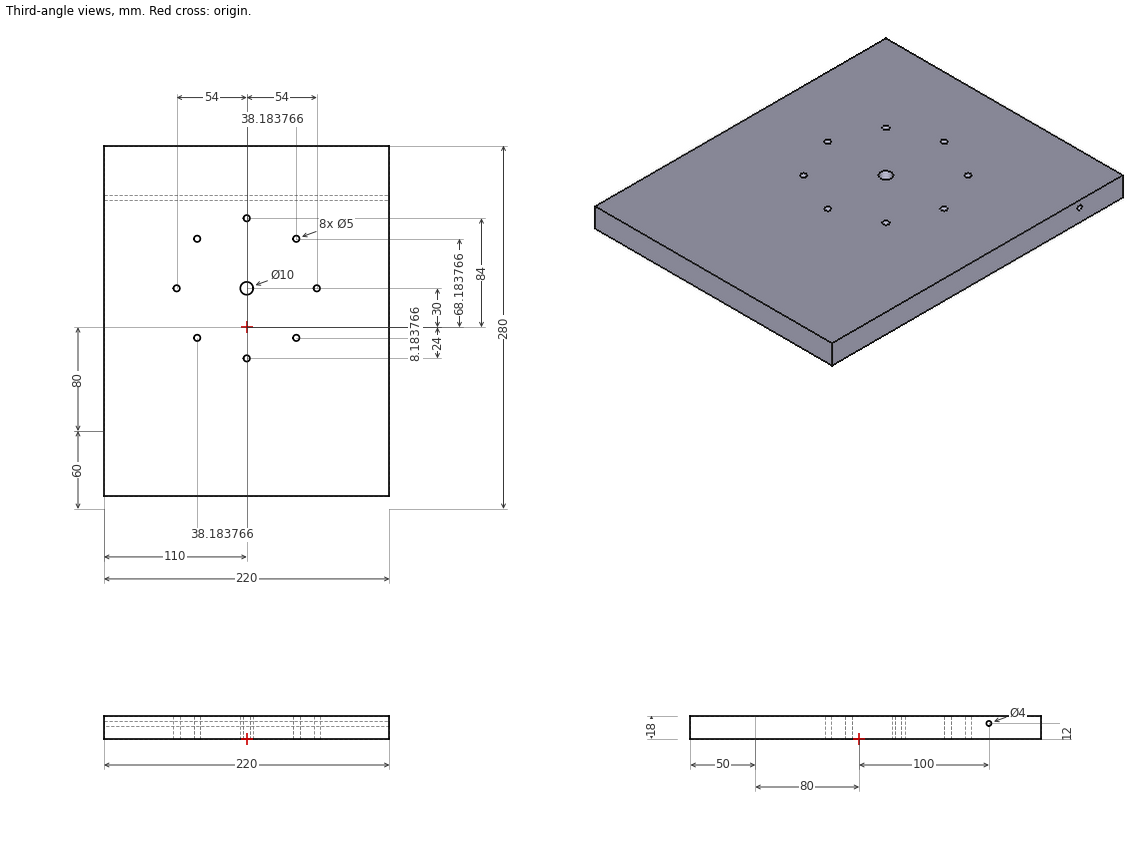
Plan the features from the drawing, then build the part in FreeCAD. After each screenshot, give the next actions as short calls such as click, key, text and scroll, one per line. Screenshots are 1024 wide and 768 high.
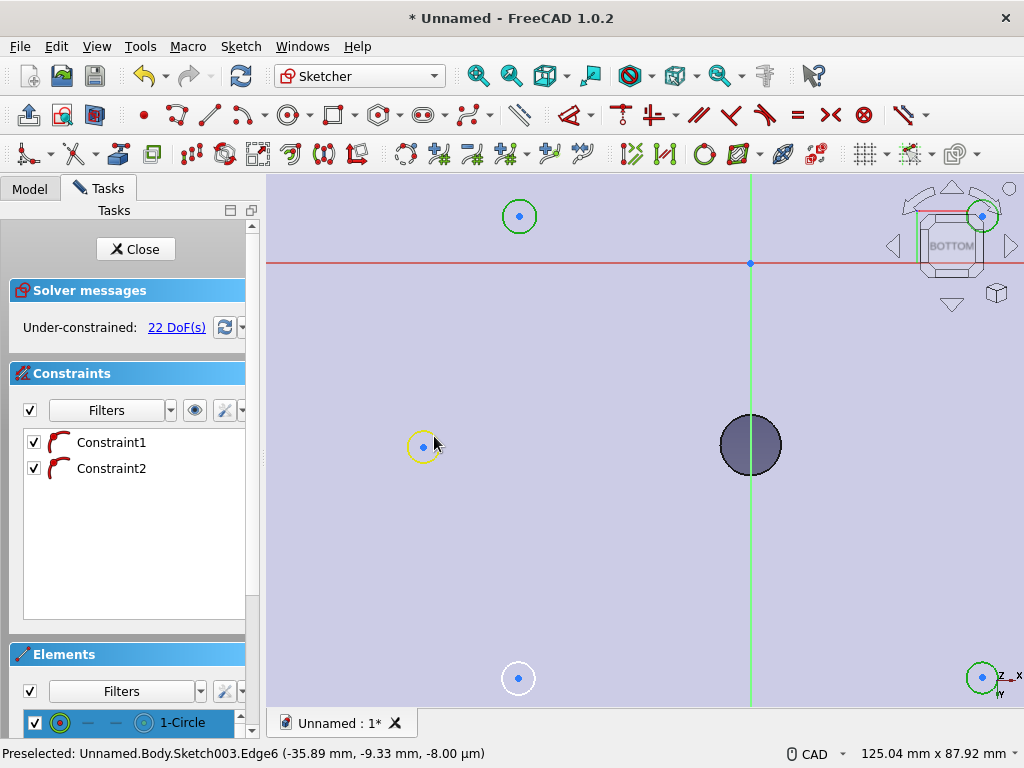
click(435, 436)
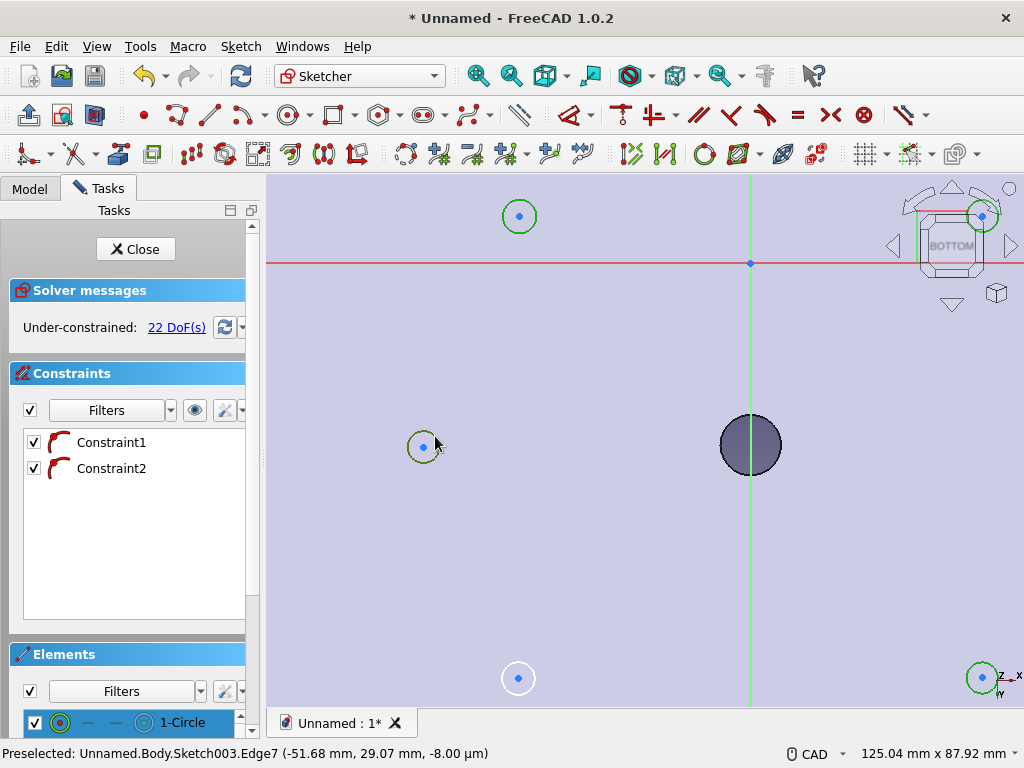
click(530, 667)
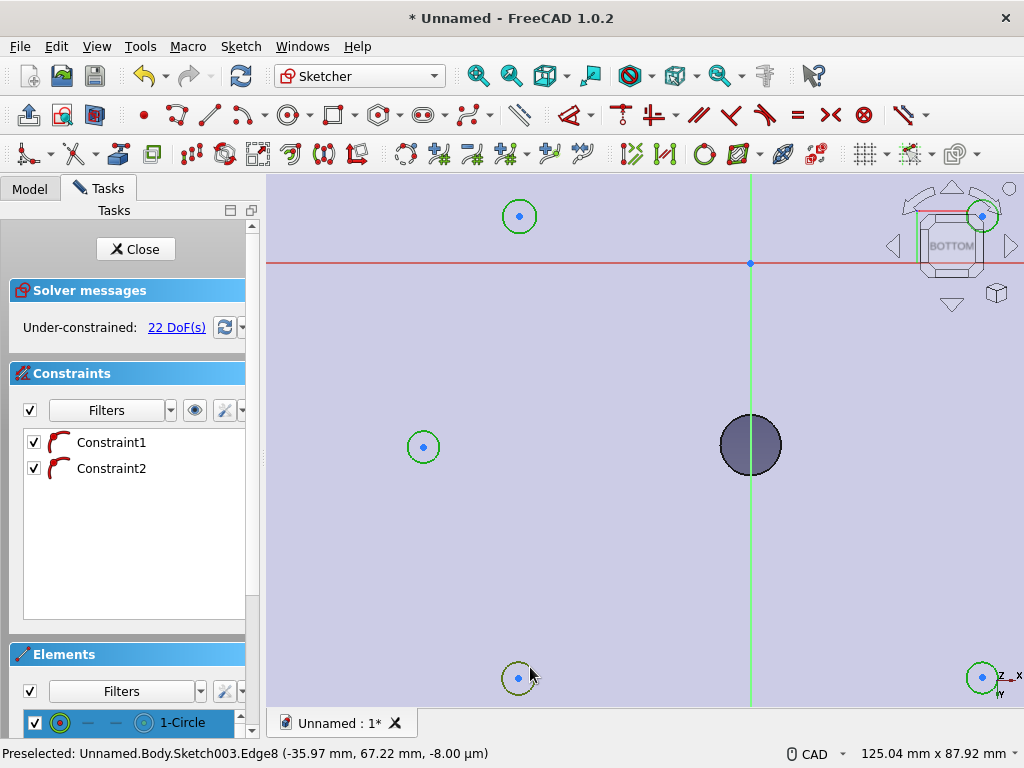
click(798, 116)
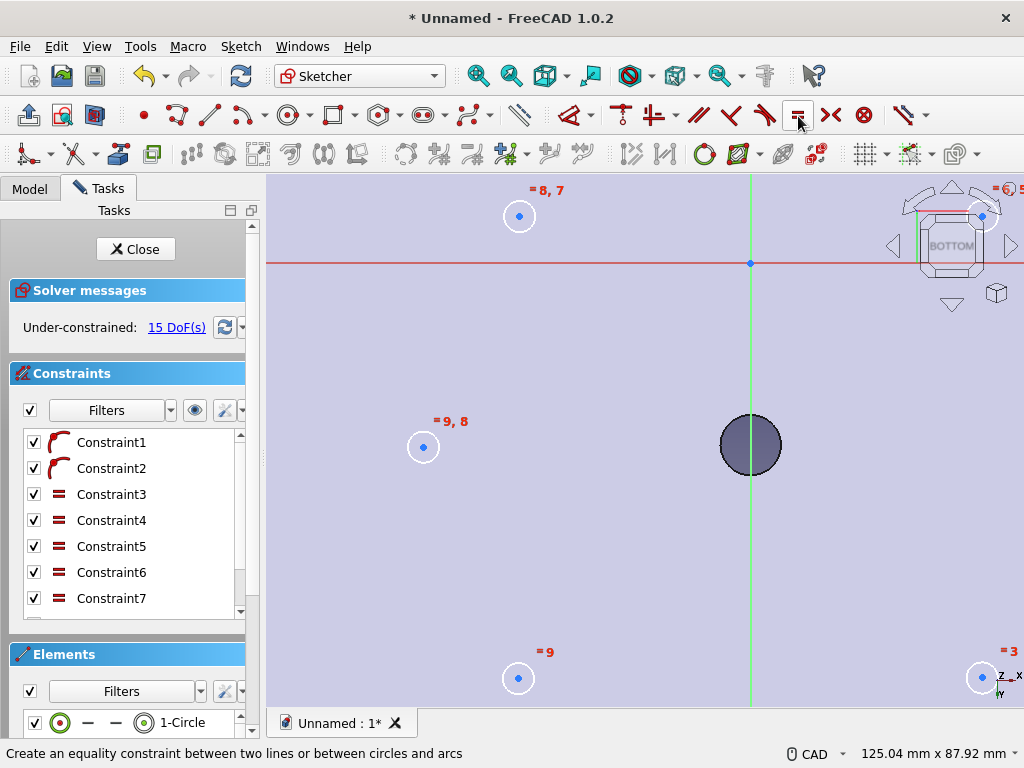
scroll(434, 437, down, 4)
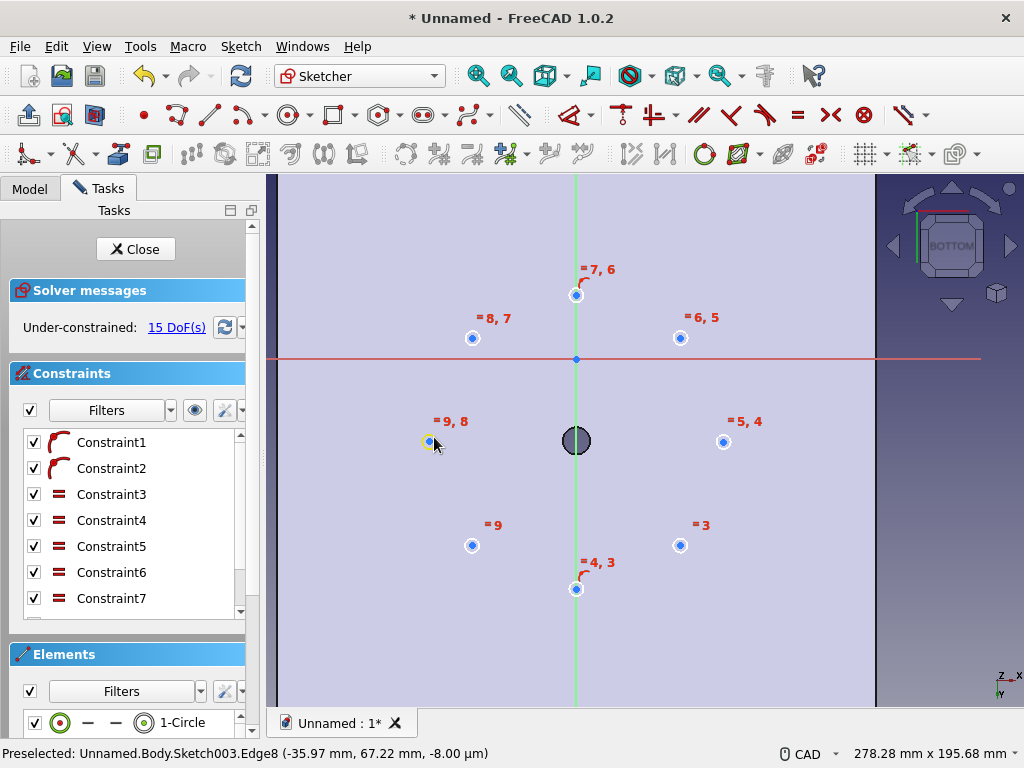
click(680, 546)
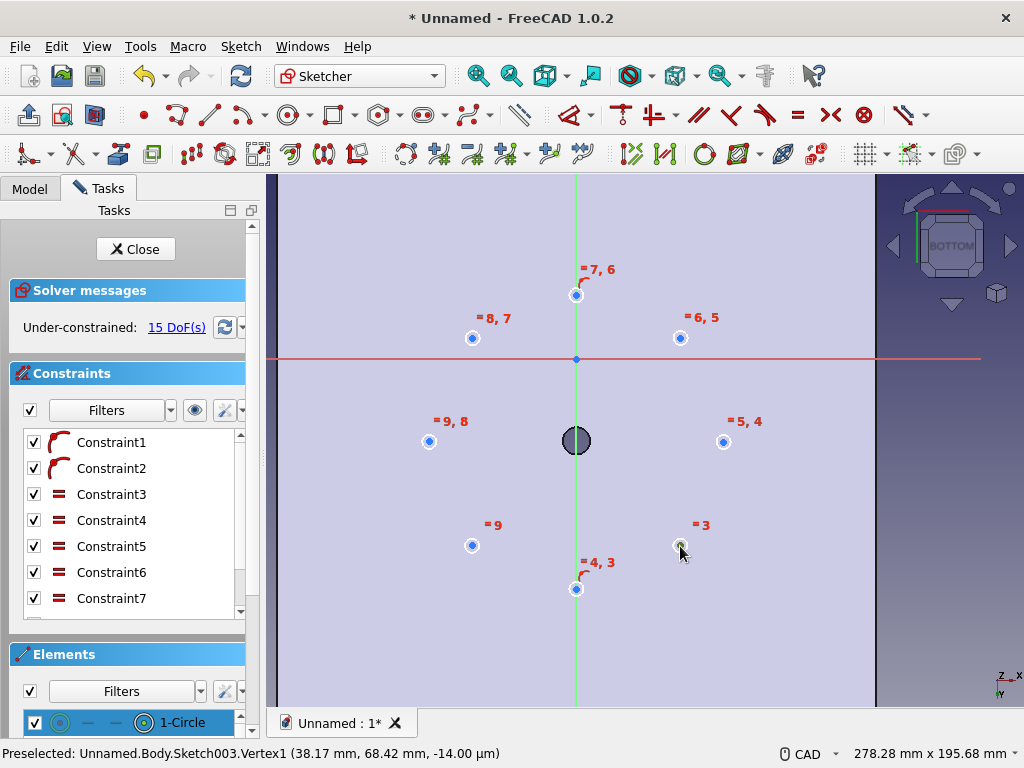
click(681, 338)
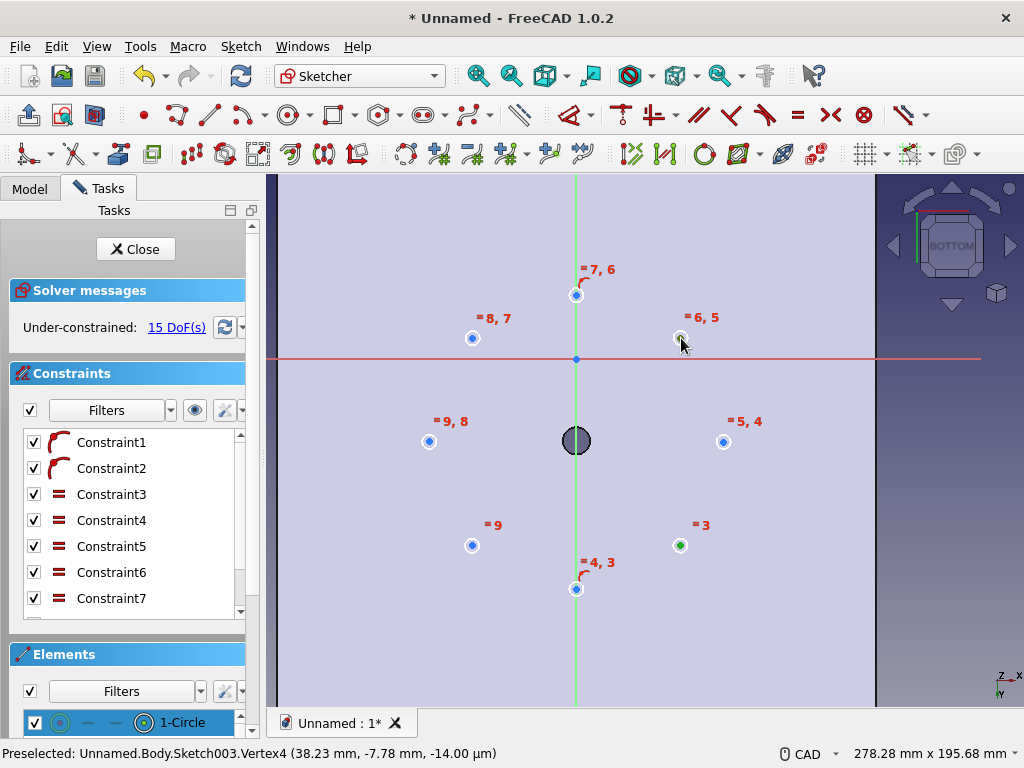
key(v)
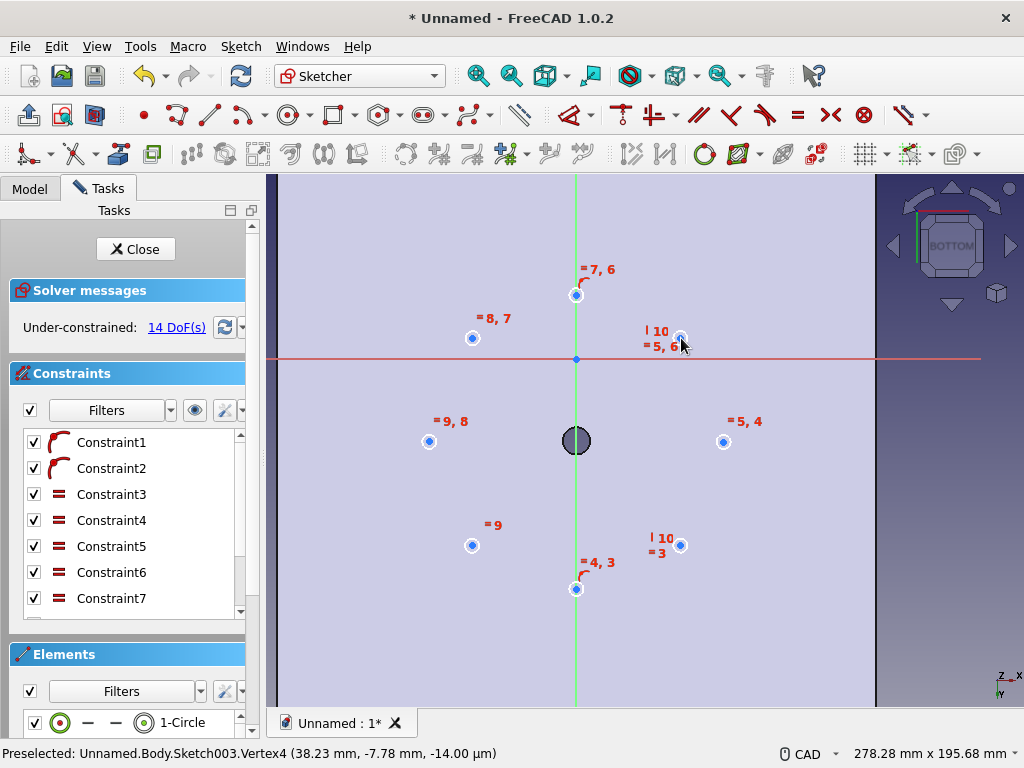
click(680, 338)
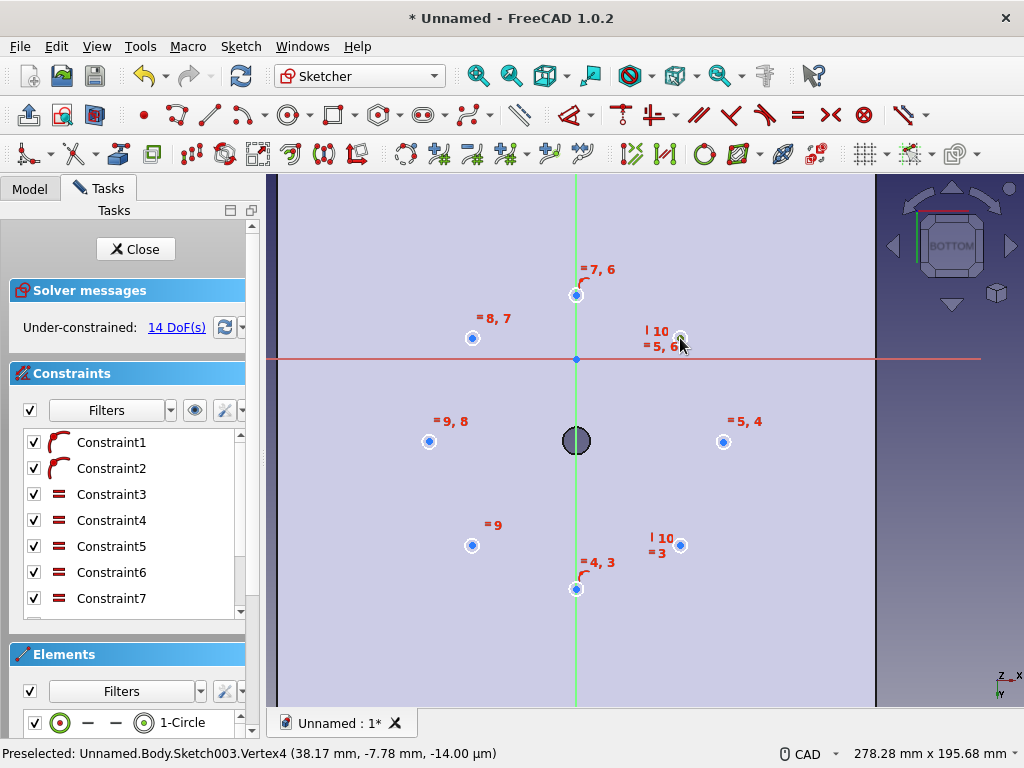
click(473, 338)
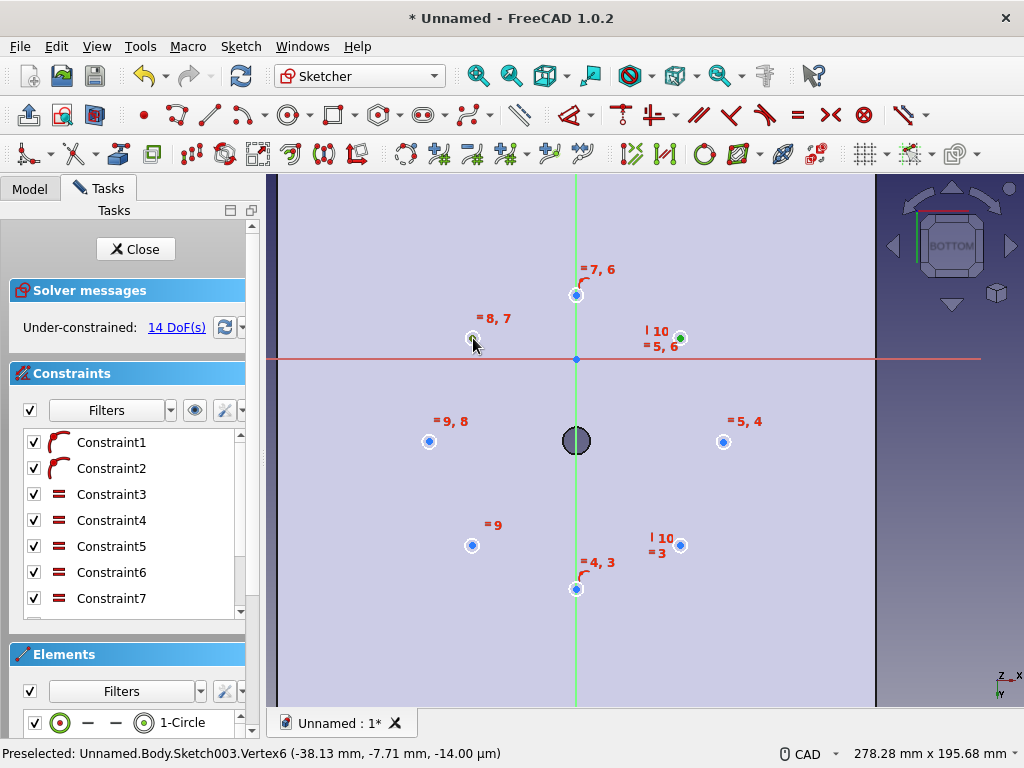
key(h)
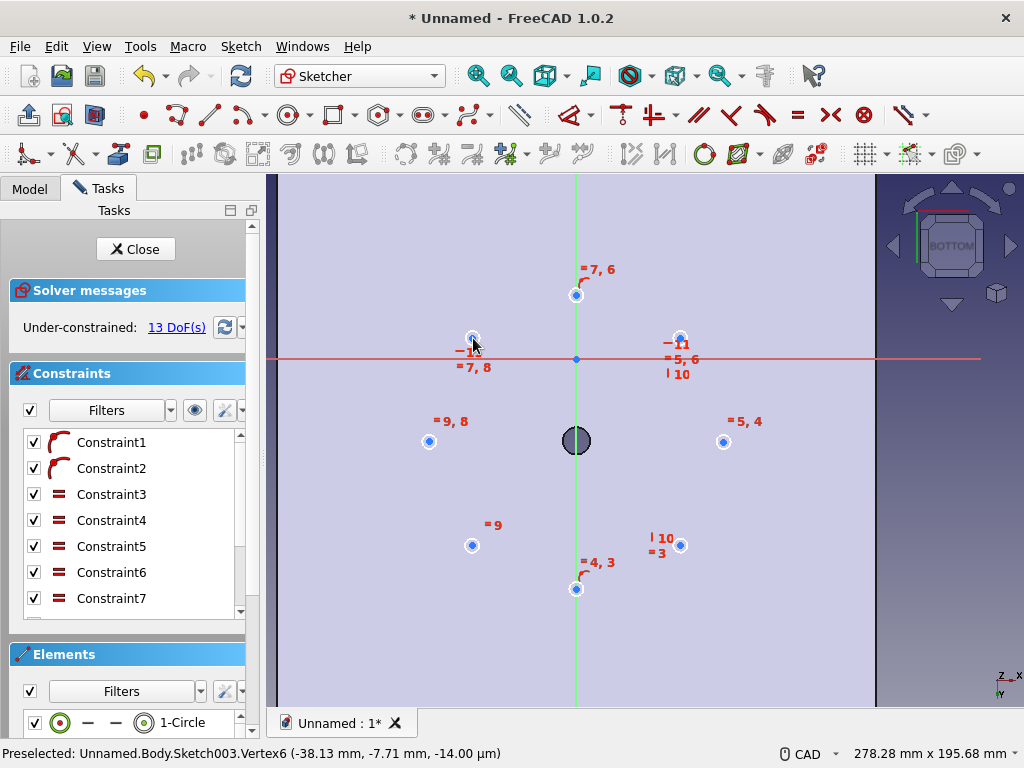
click(724, 442)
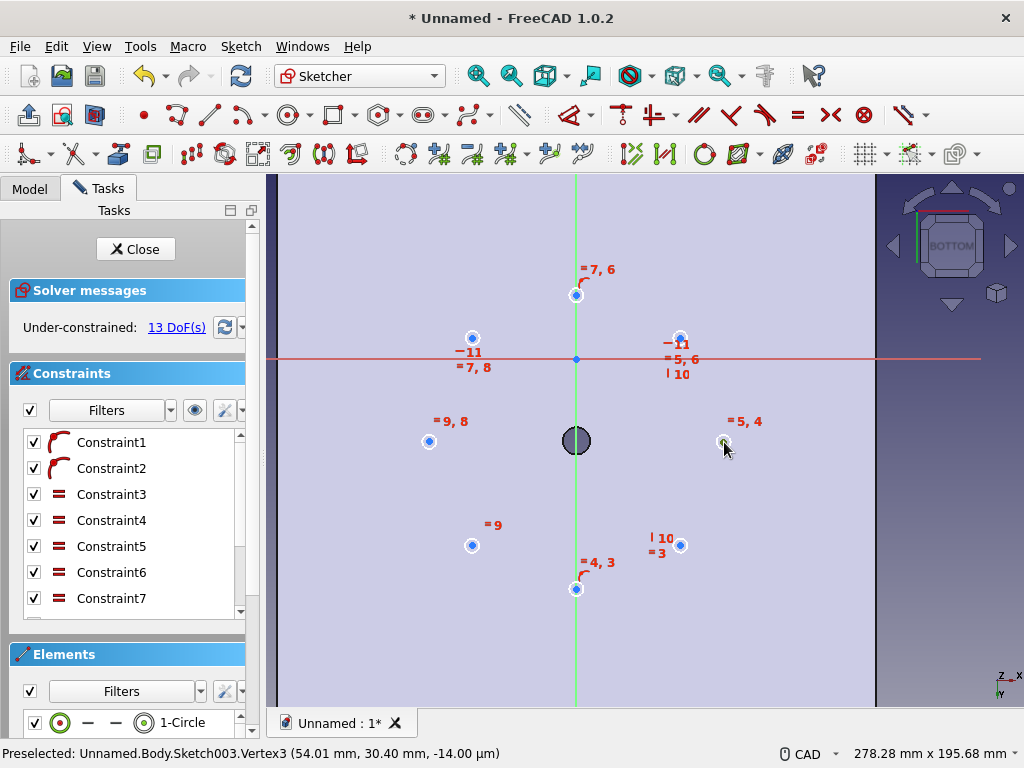
click(429, 442)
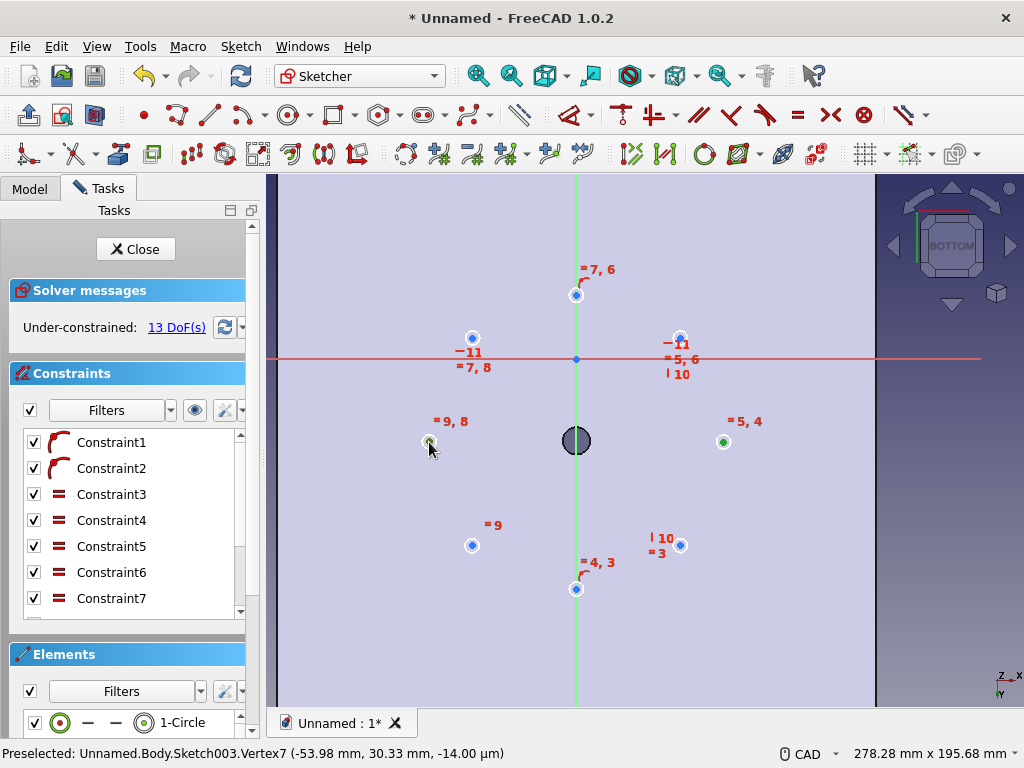
key(h)